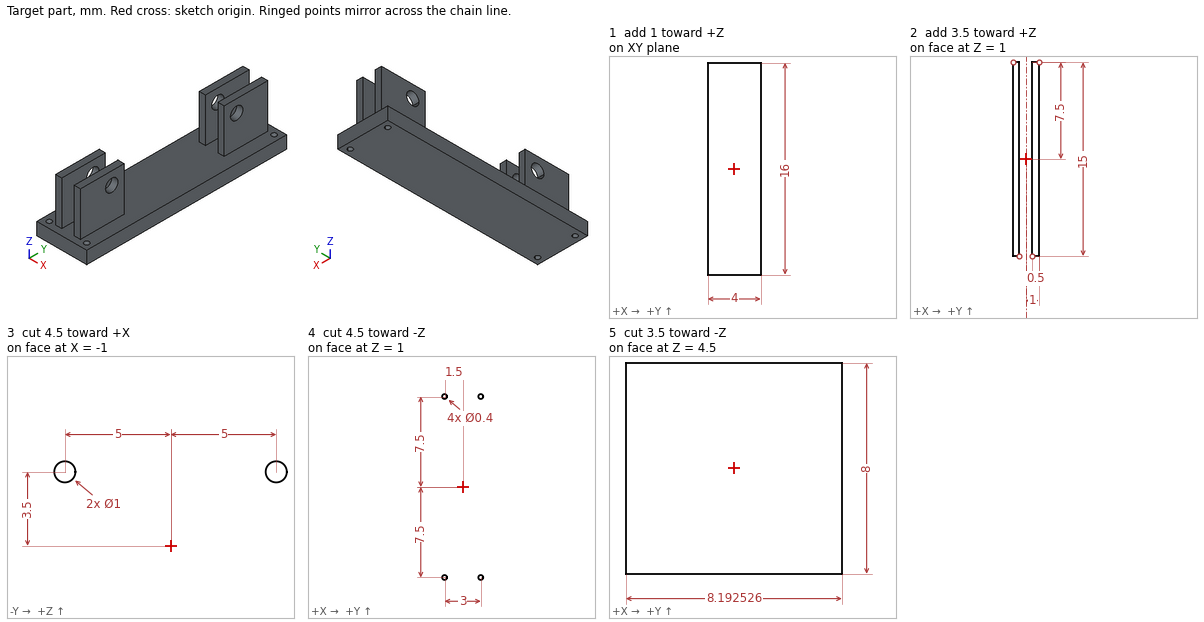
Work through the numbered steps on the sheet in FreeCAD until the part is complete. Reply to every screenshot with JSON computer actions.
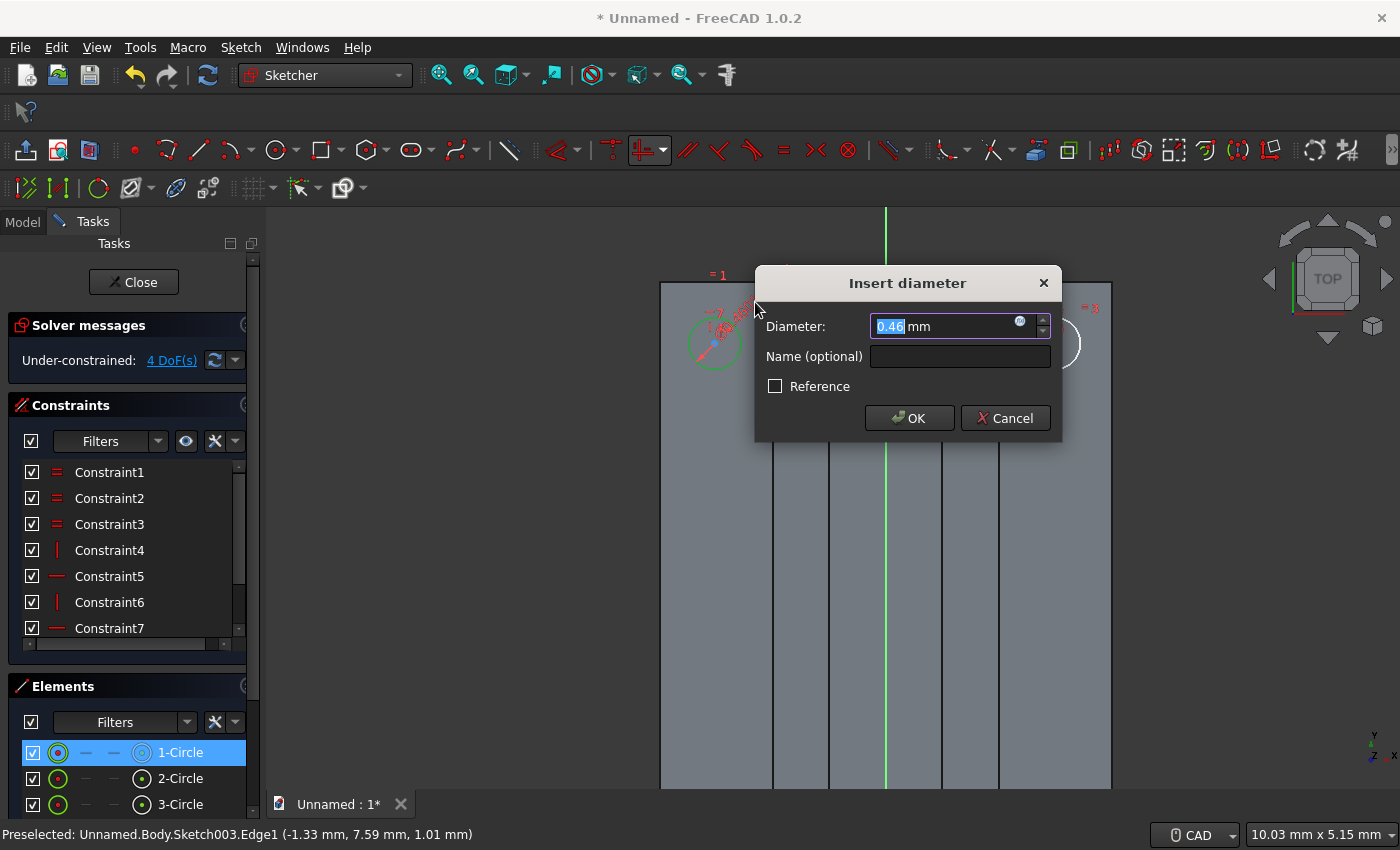
{"action": "type", "text": "0.4"}
{"action": "key", "text": "Return"}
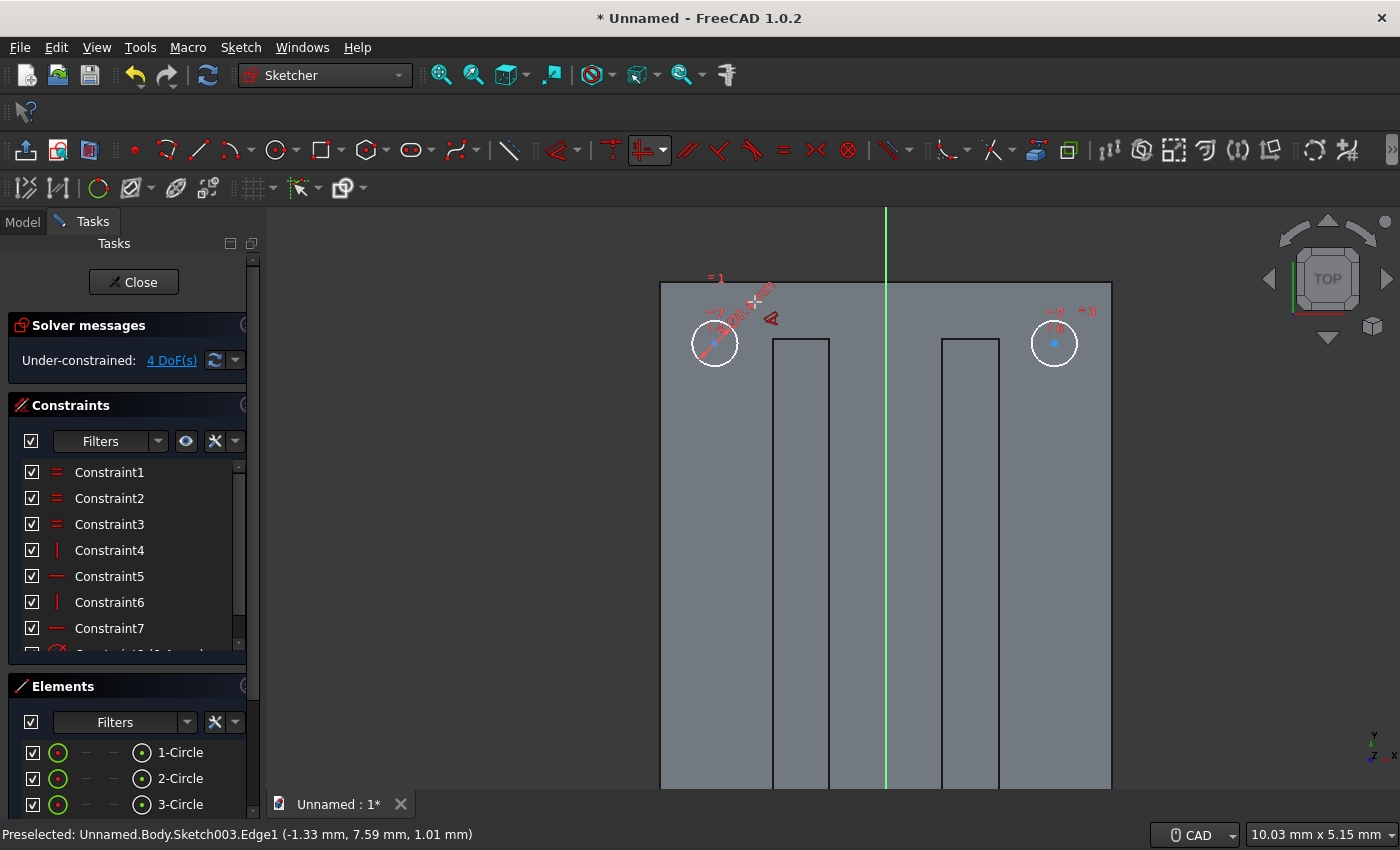
{"action": "scroll", "coordinate": [734, 324], "scroll_direction": "down", "scroll_amount": 8}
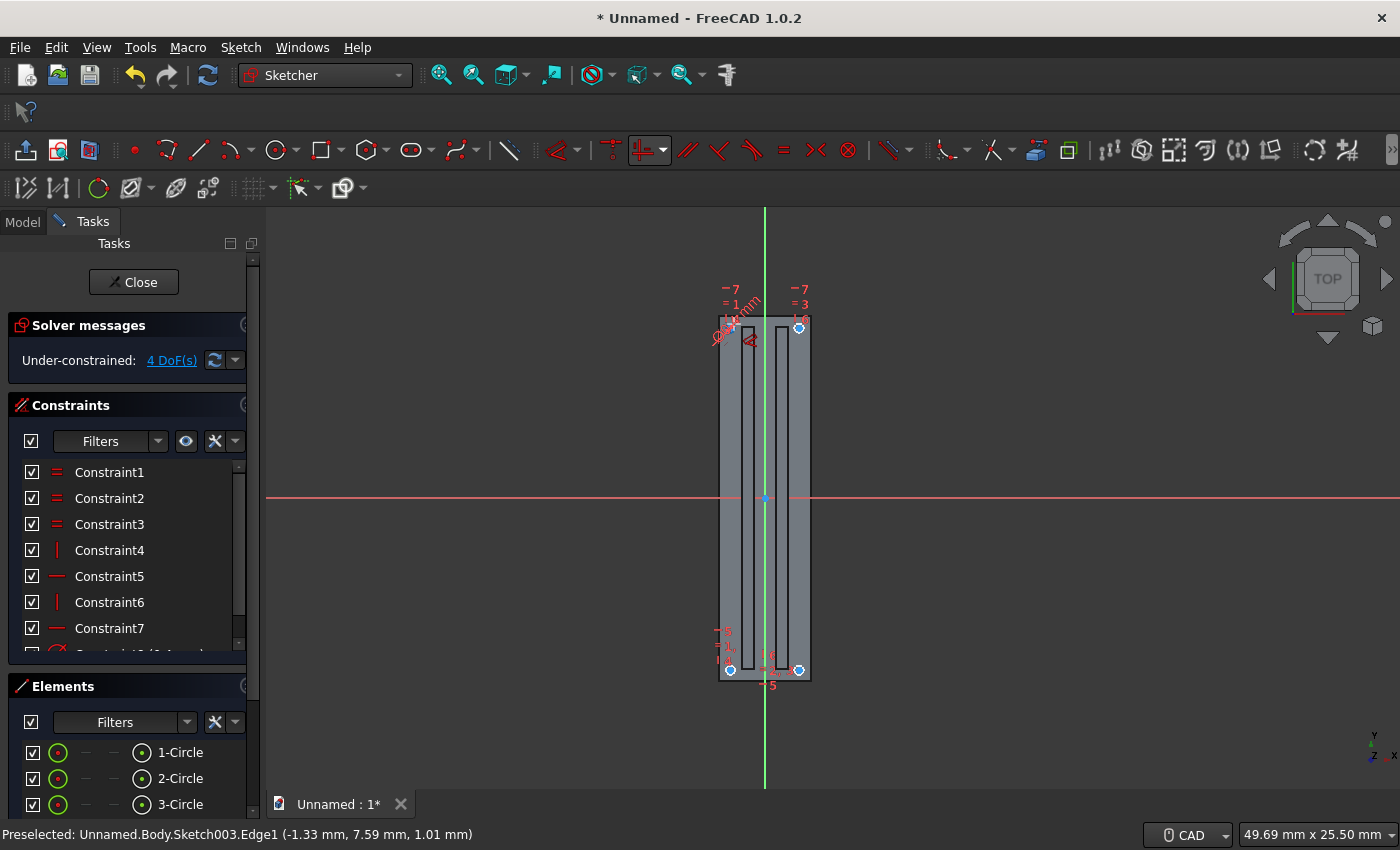
{"action": "left_click", "coordinate": [730, 670]}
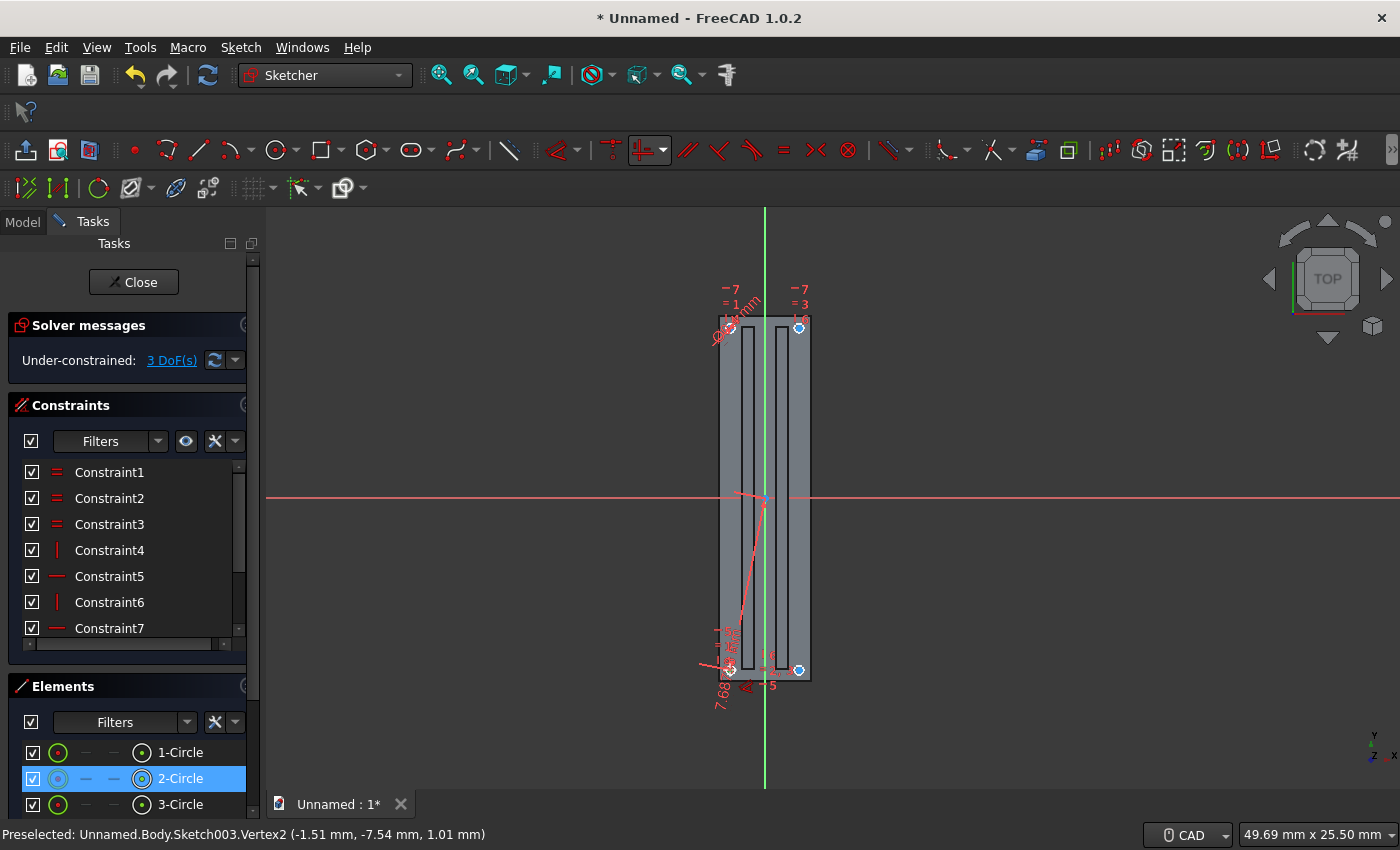
{"action": "left_click", "coordinate": [799, 670]}
{"action": "left_click", "coordinate": [749, 704]}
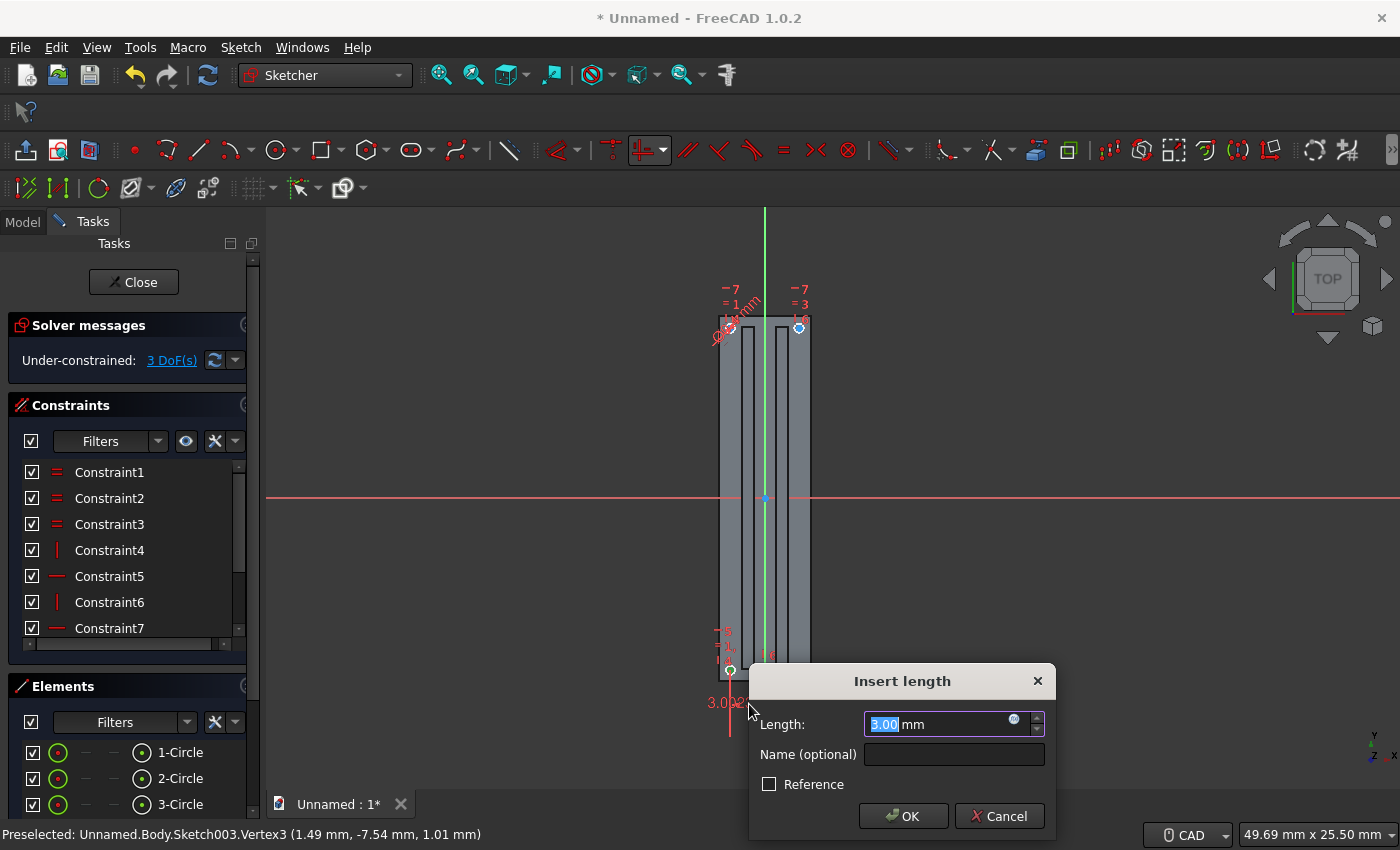
{"action": "type", "text": "3"}
{"action": "key", "text": "Return"}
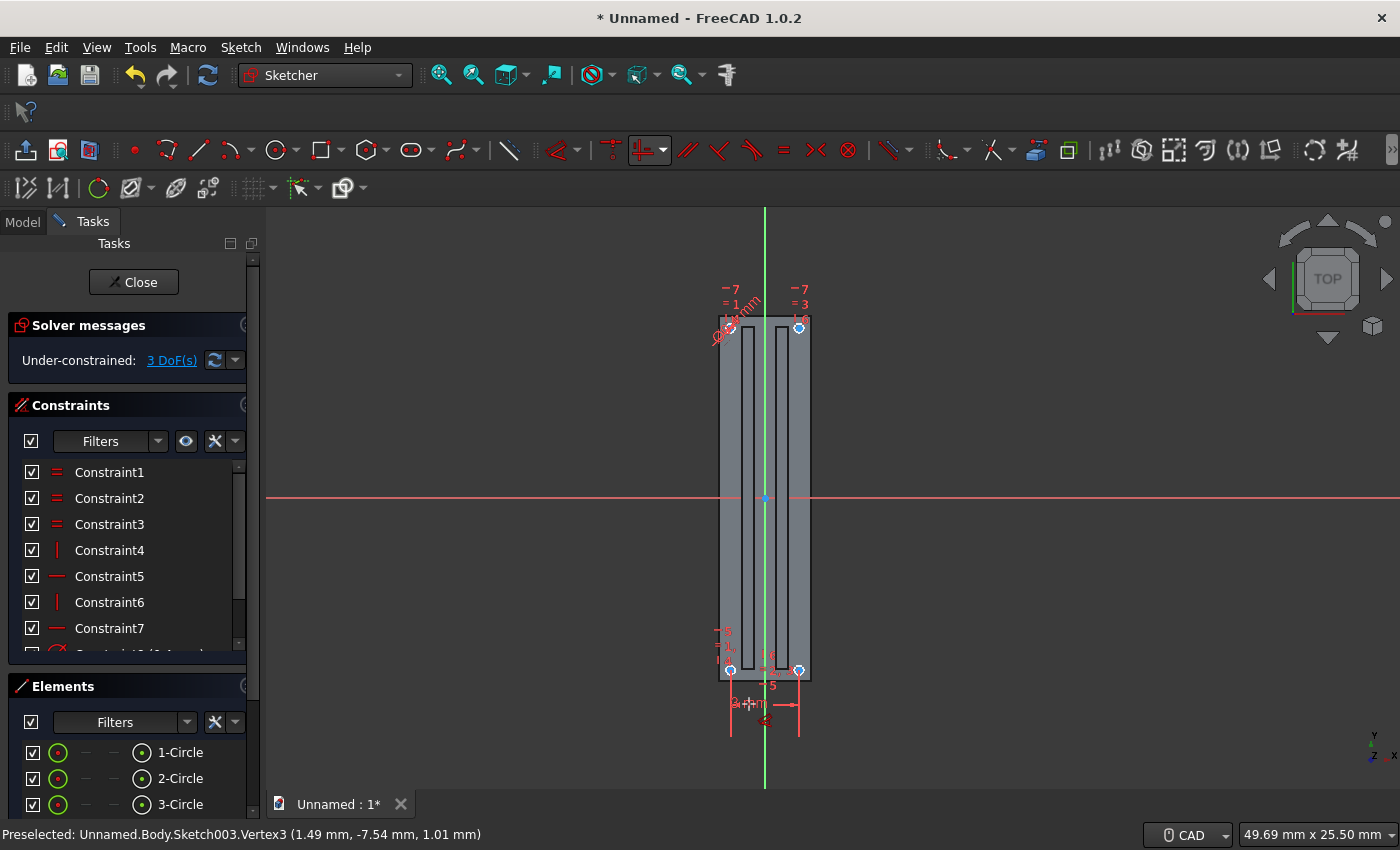
{"action": "left_click", "coordinate": [731, 328]}
{"action": "left_click", "coordinate": [748, 294]}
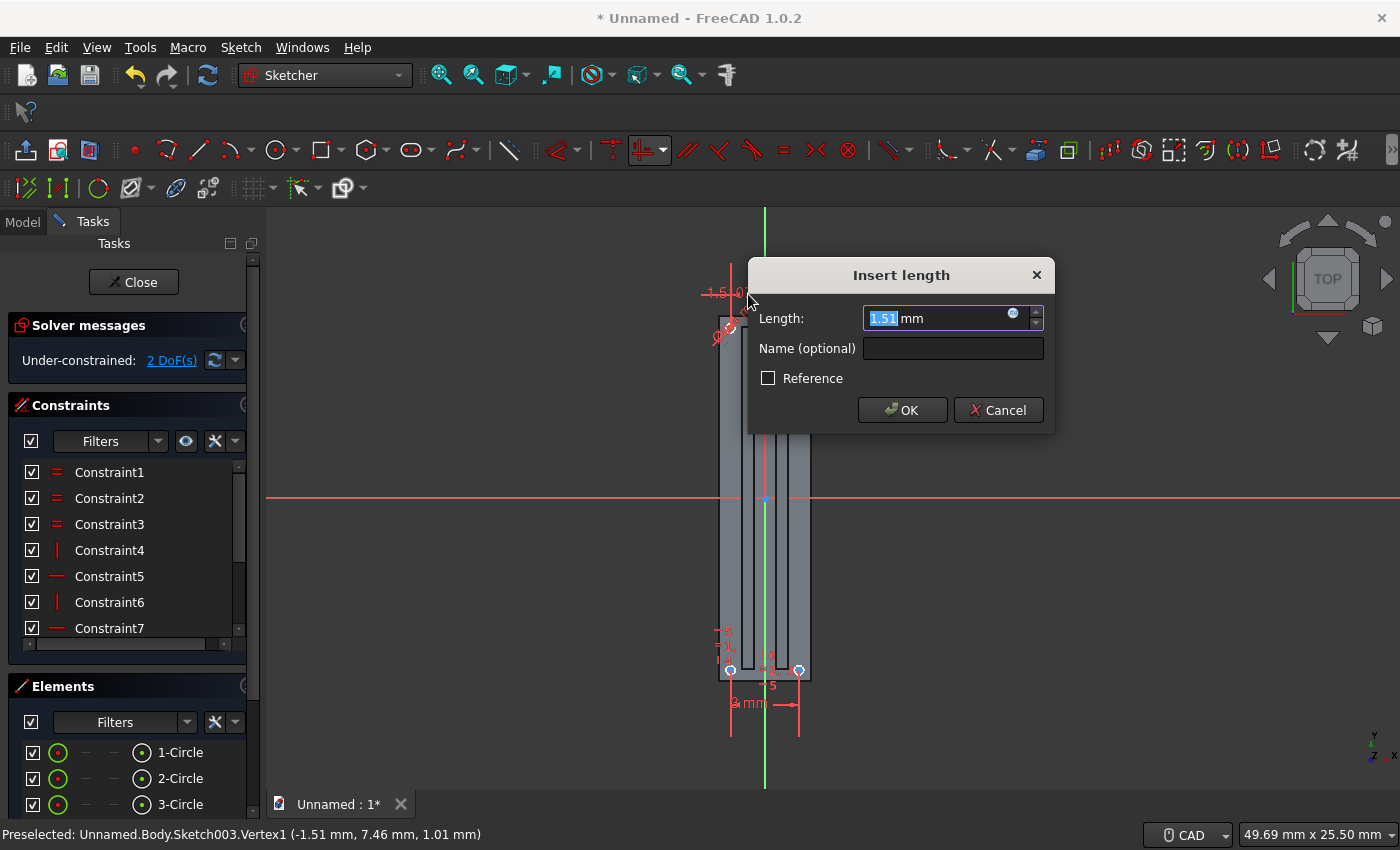
{"action": "type", "text": "1.5"}
{"action": "key", "text": "Return"}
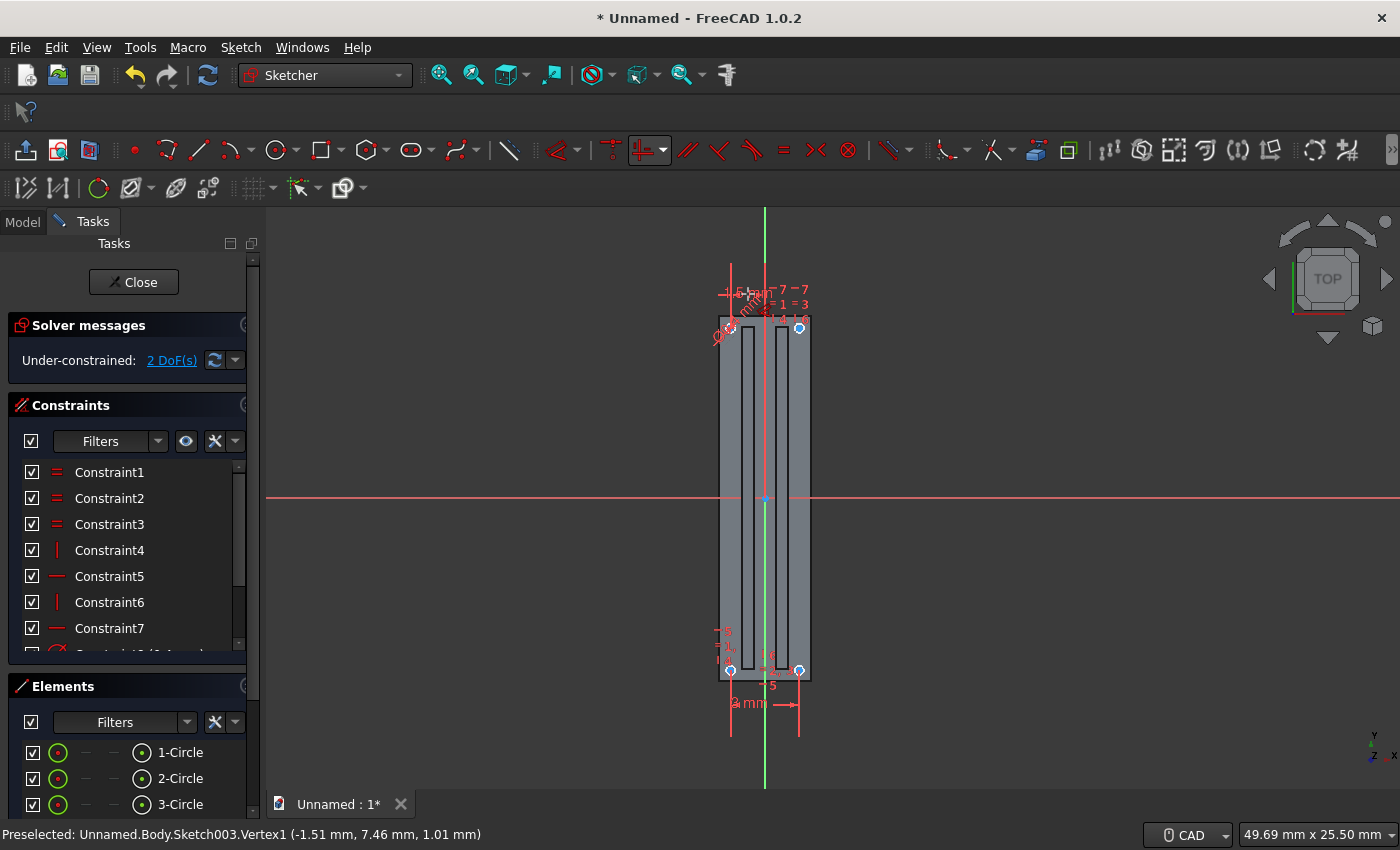
{"action": "left_click", "coordinate": [731, 328]}
{"action": "left_click", "coordinate": [697, 413]}